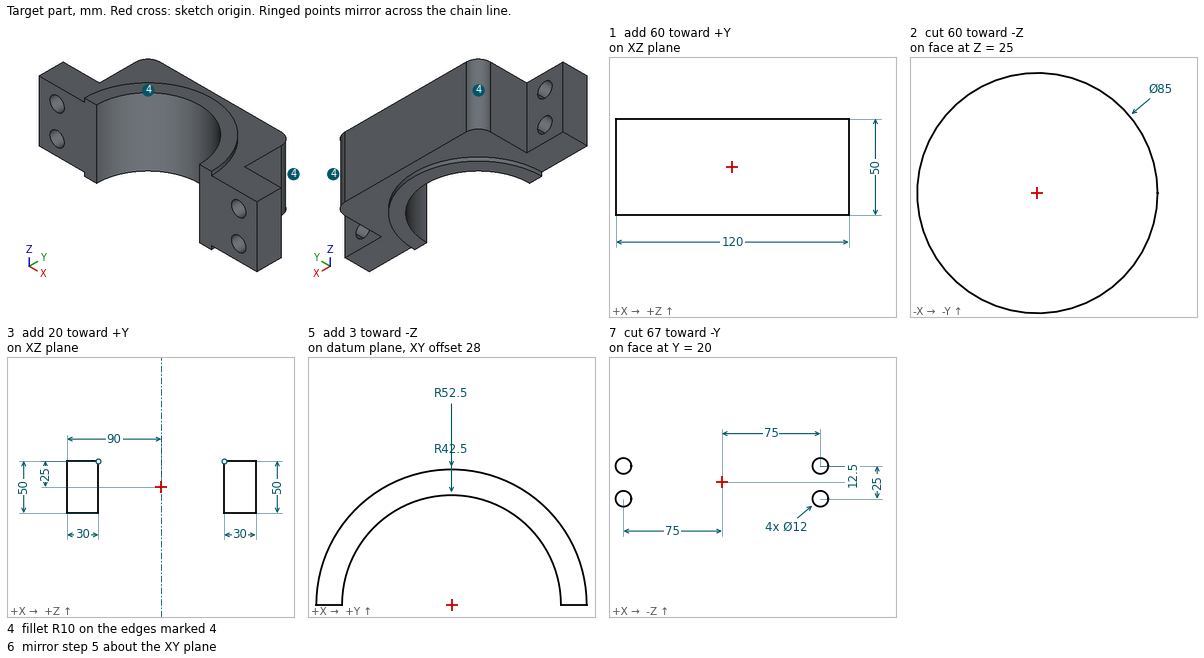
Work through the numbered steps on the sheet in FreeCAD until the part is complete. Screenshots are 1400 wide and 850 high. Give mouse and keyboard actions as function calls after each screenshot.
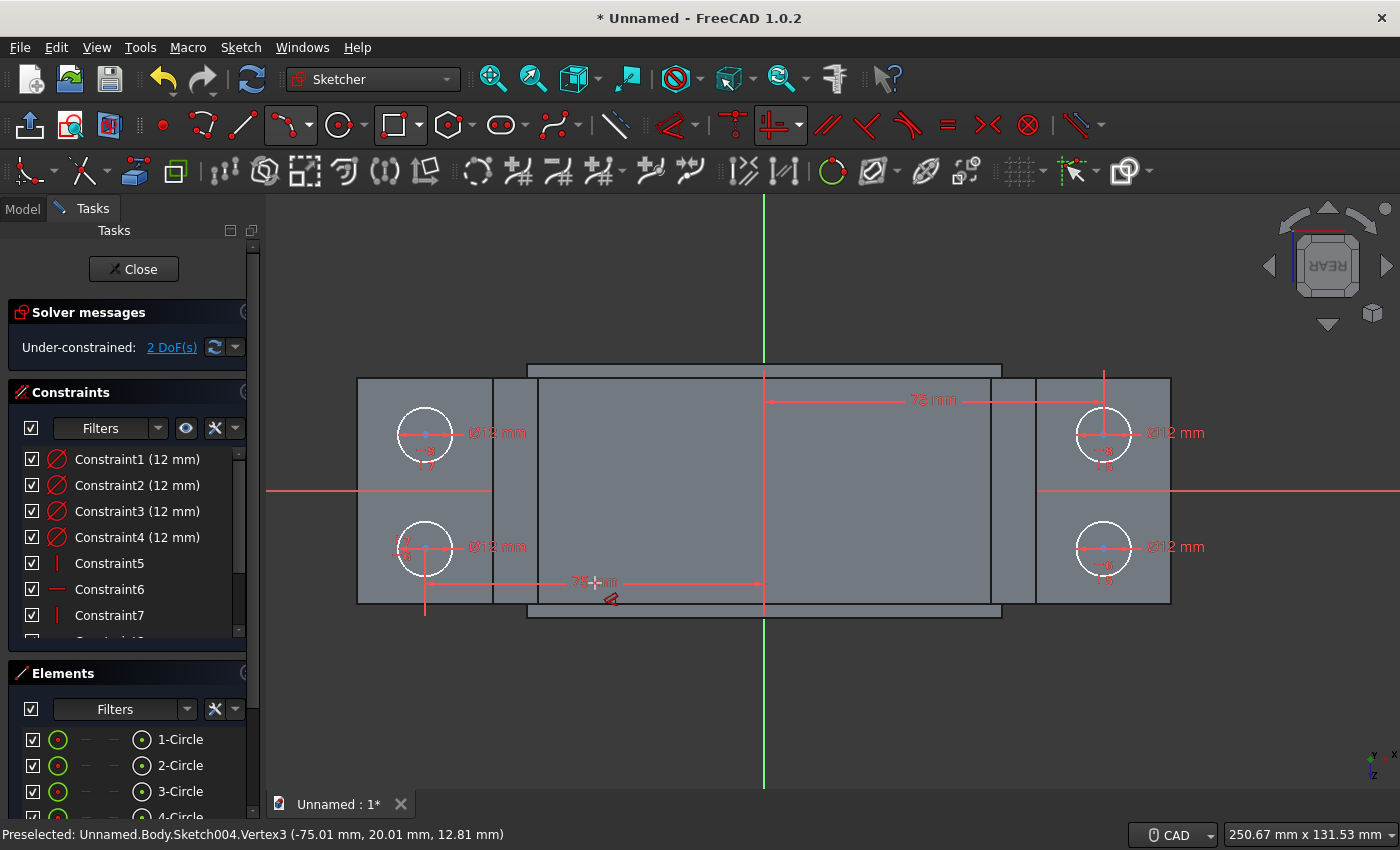
click(1104, 435)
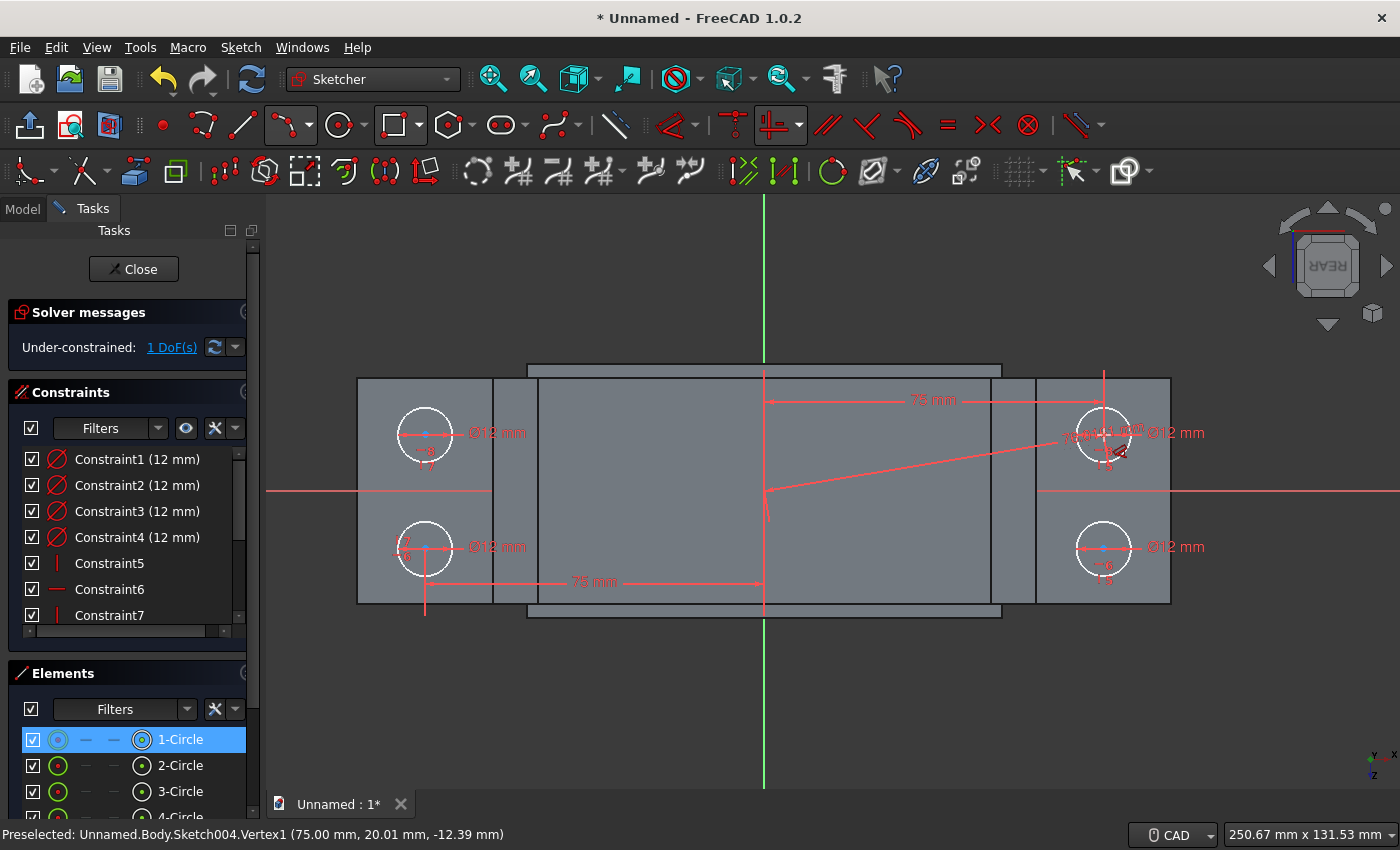
click(1104, 549)
click(1138, 466)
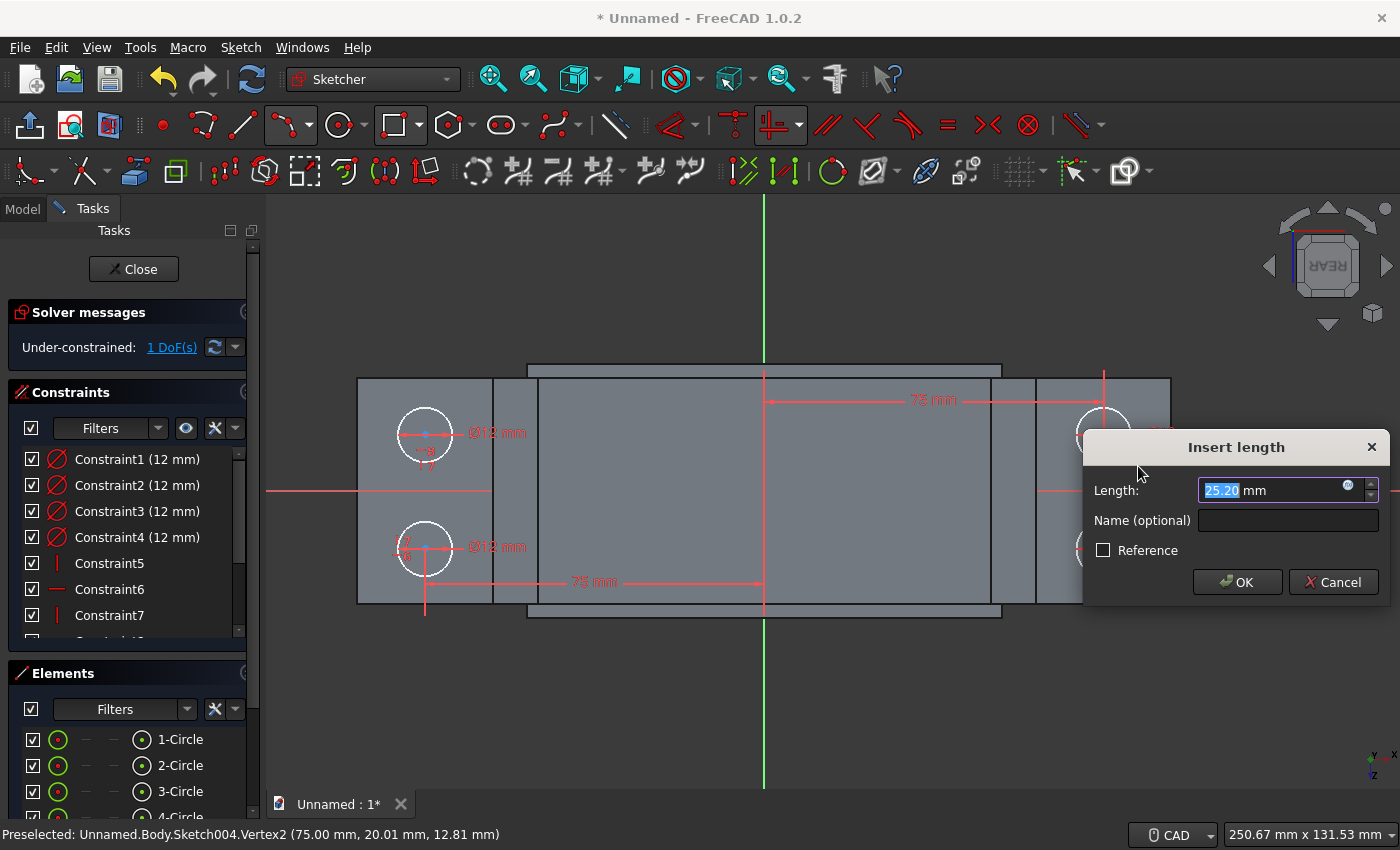
text(25)
key(Return)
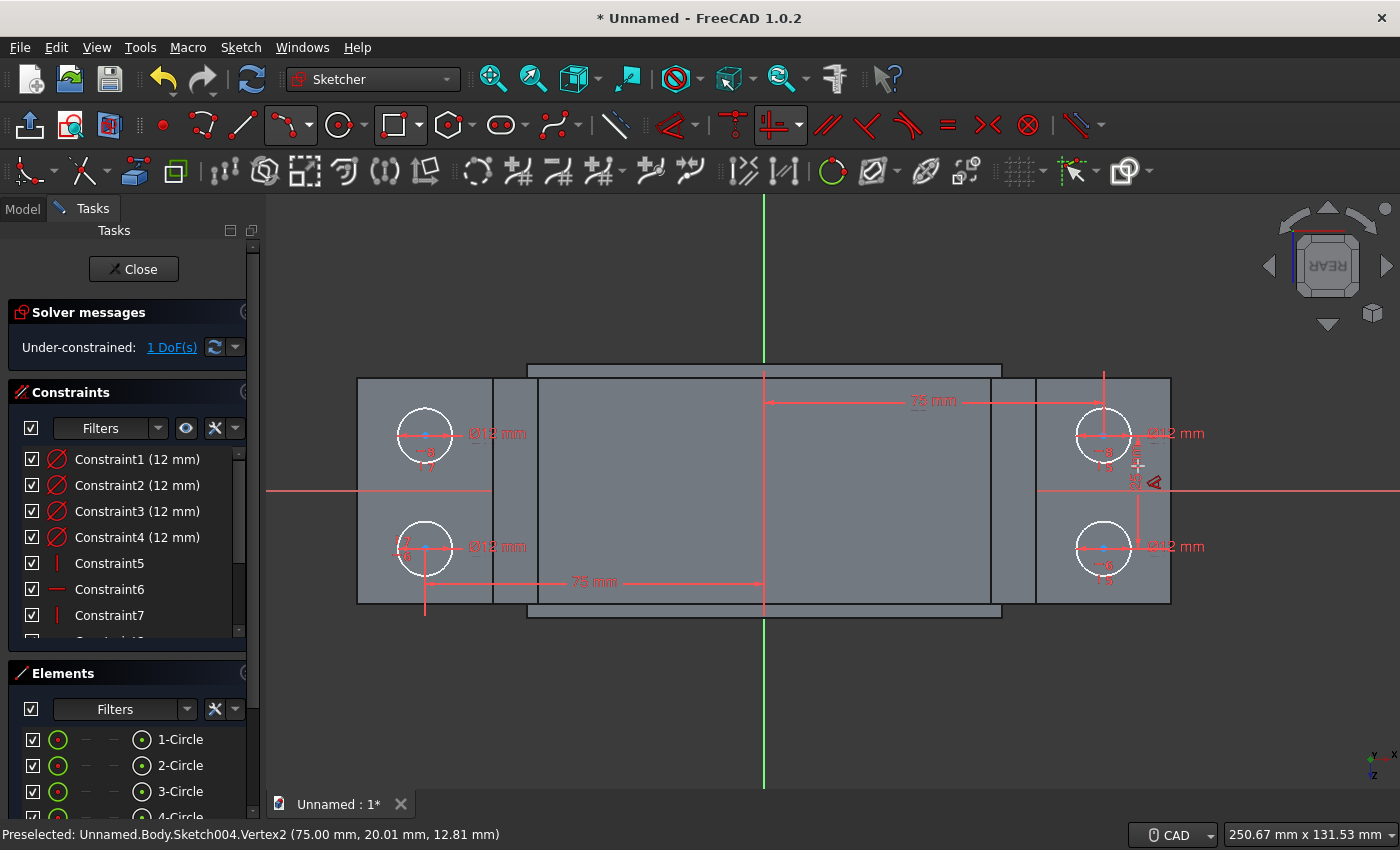
click(1104, 436)
click(730, 463)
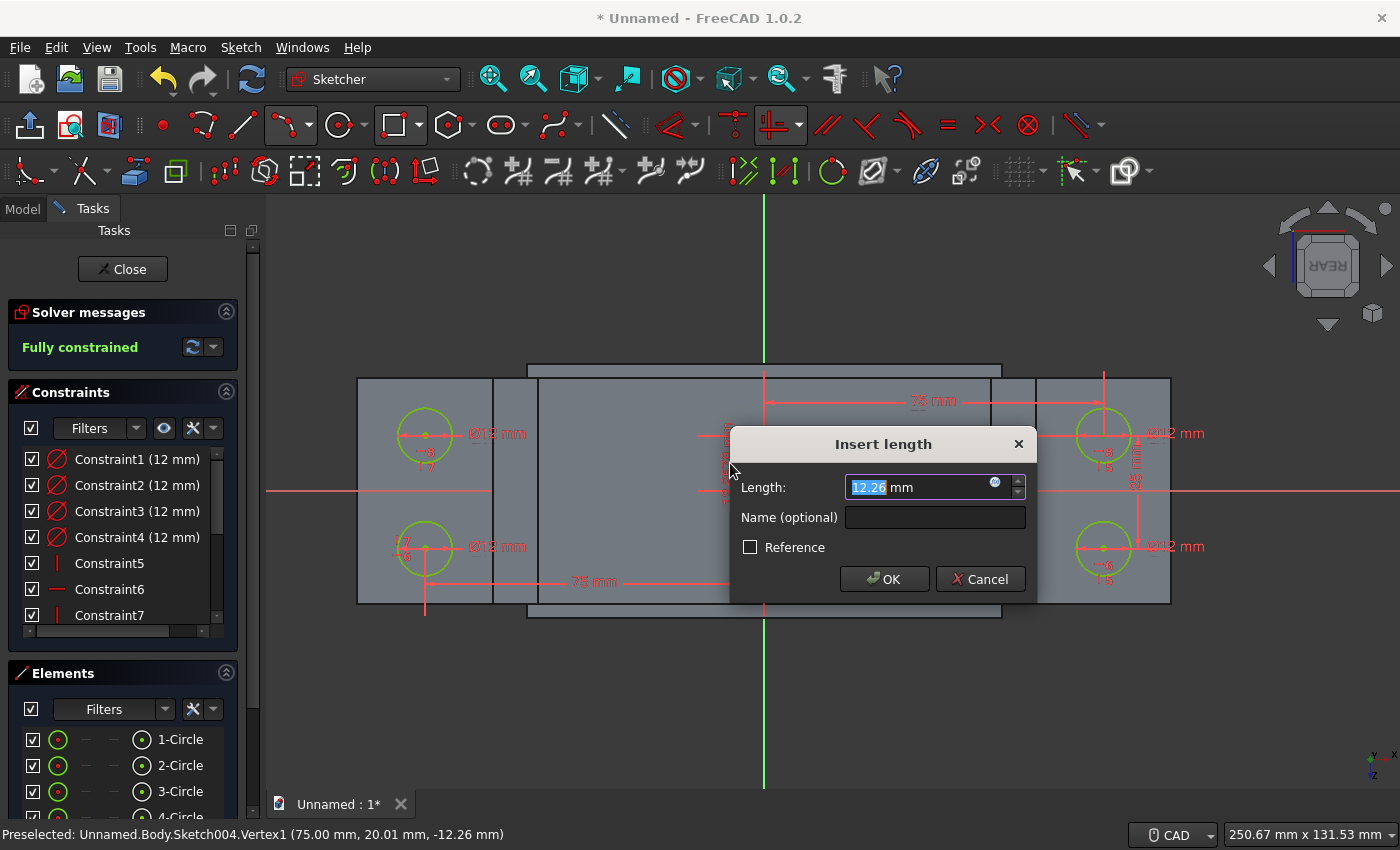
text(12.5)
key(Return)
key(Escape)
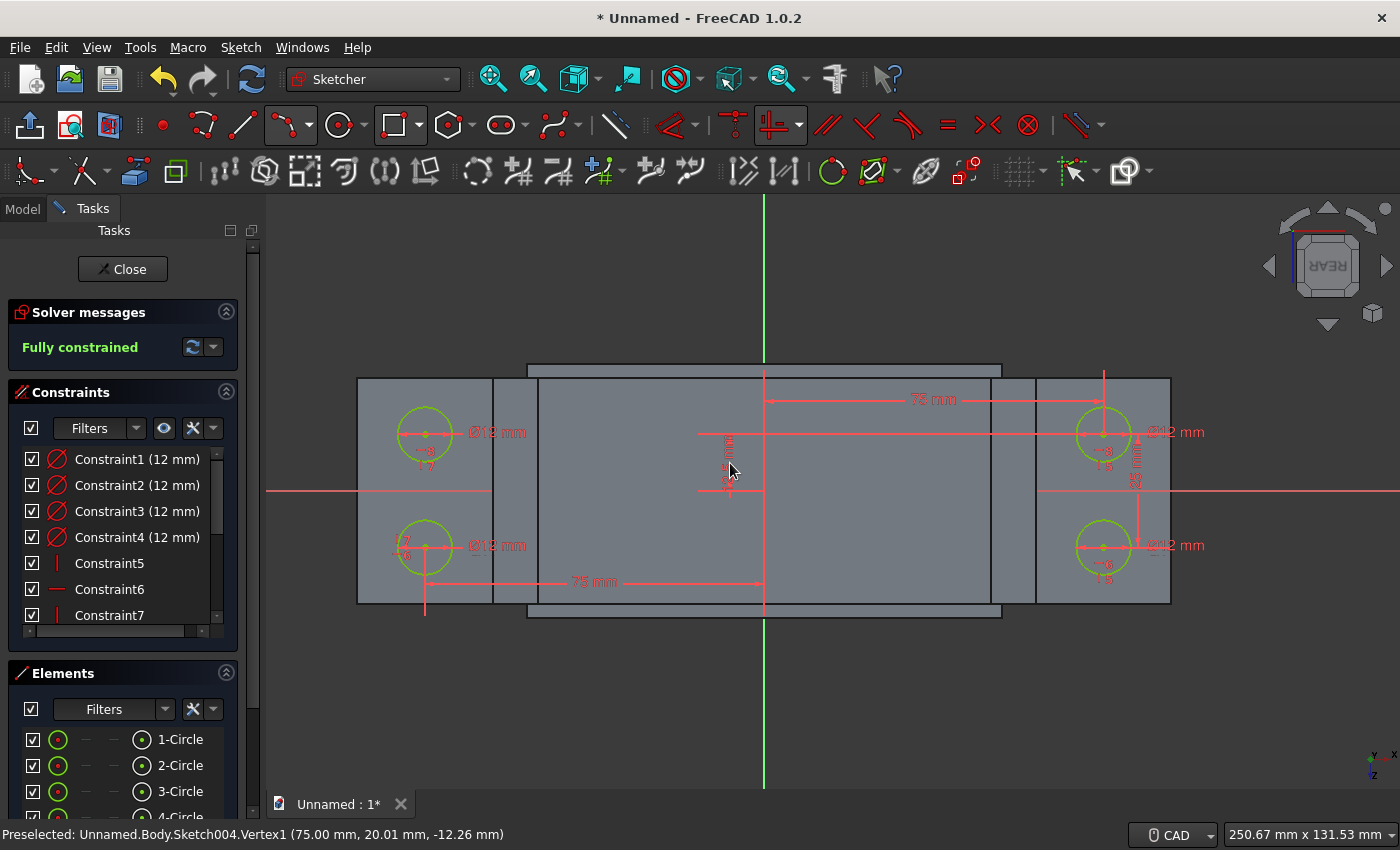
click(123, 269)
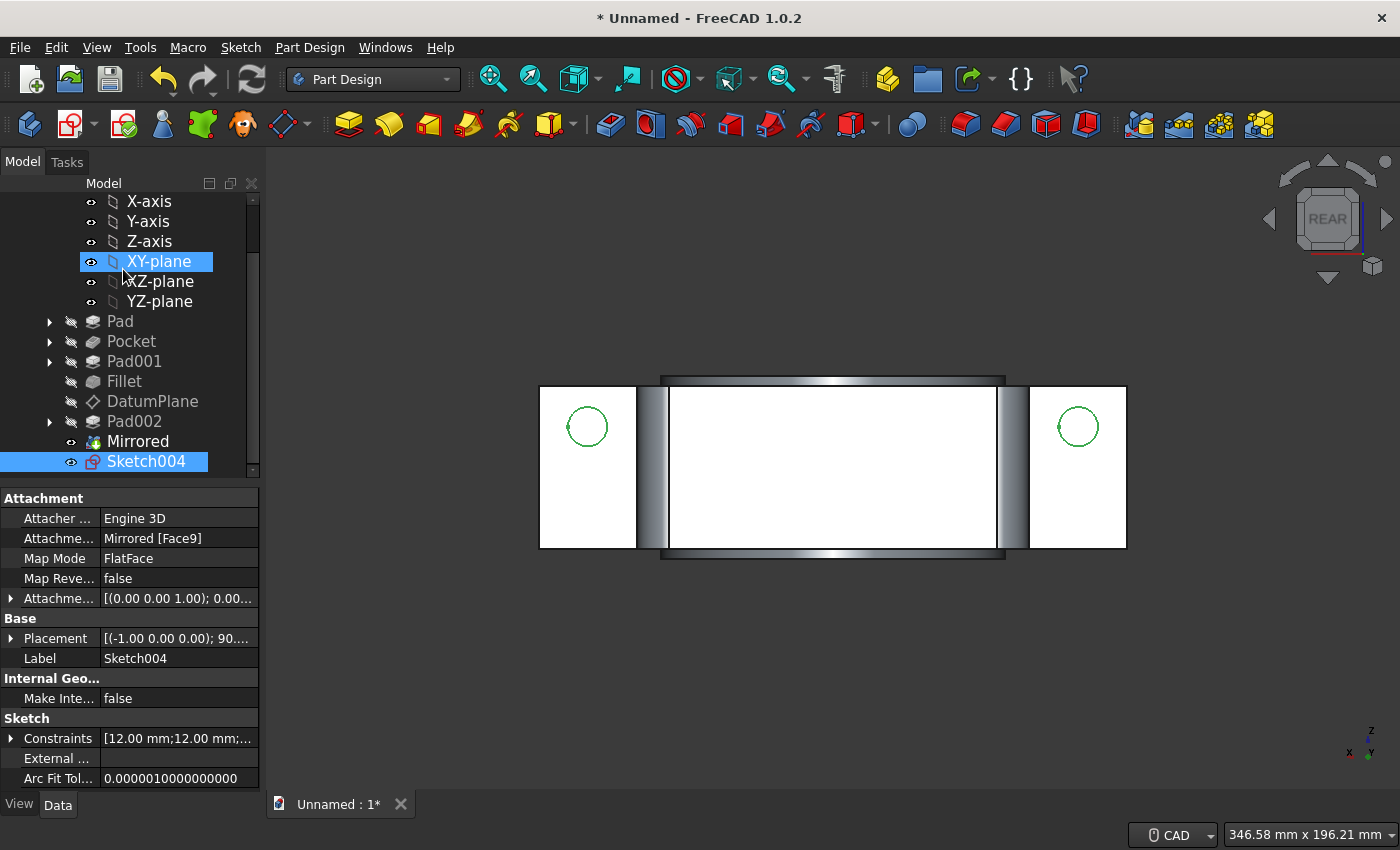
click(612, 124)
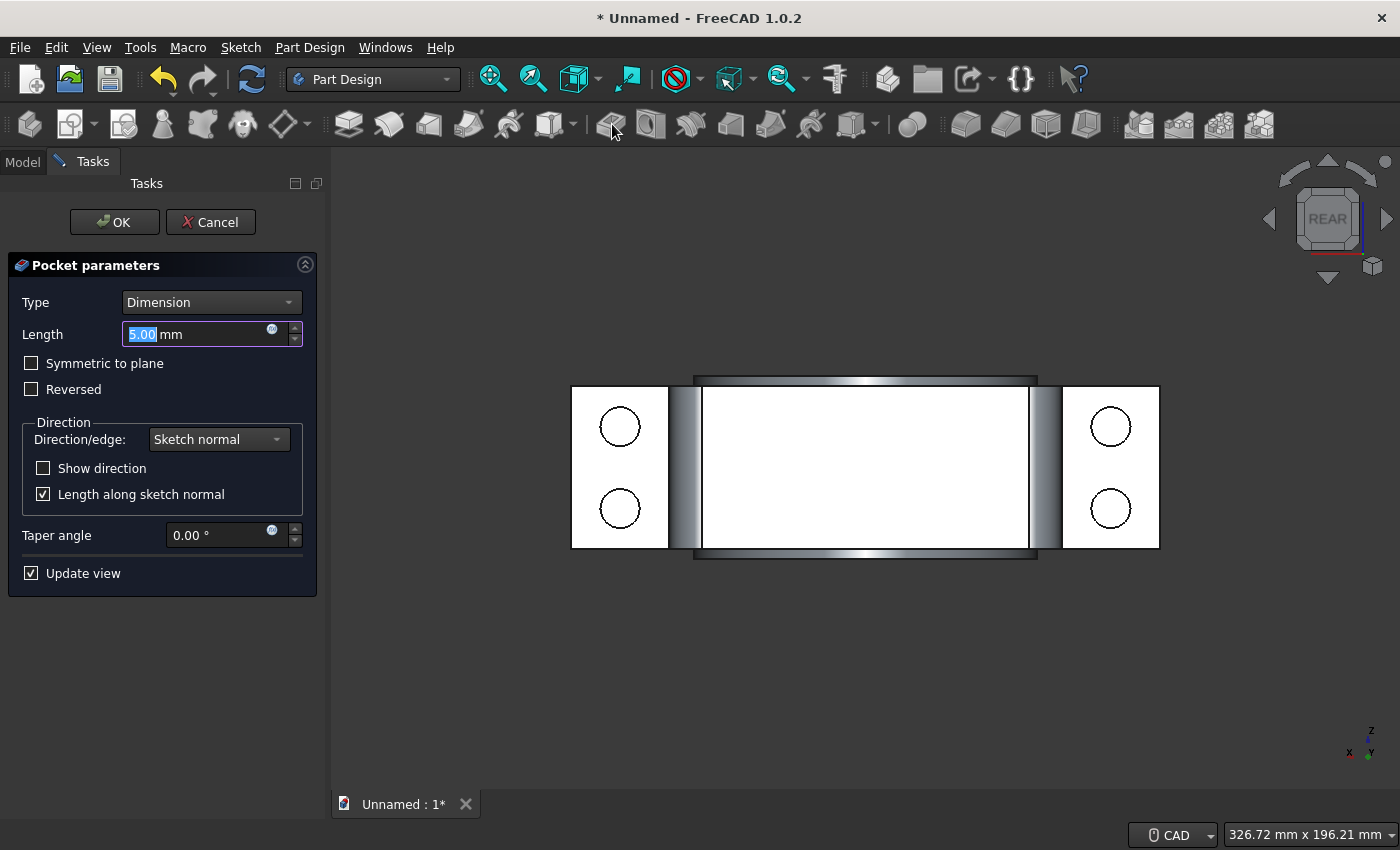
text(67)
key(Tab)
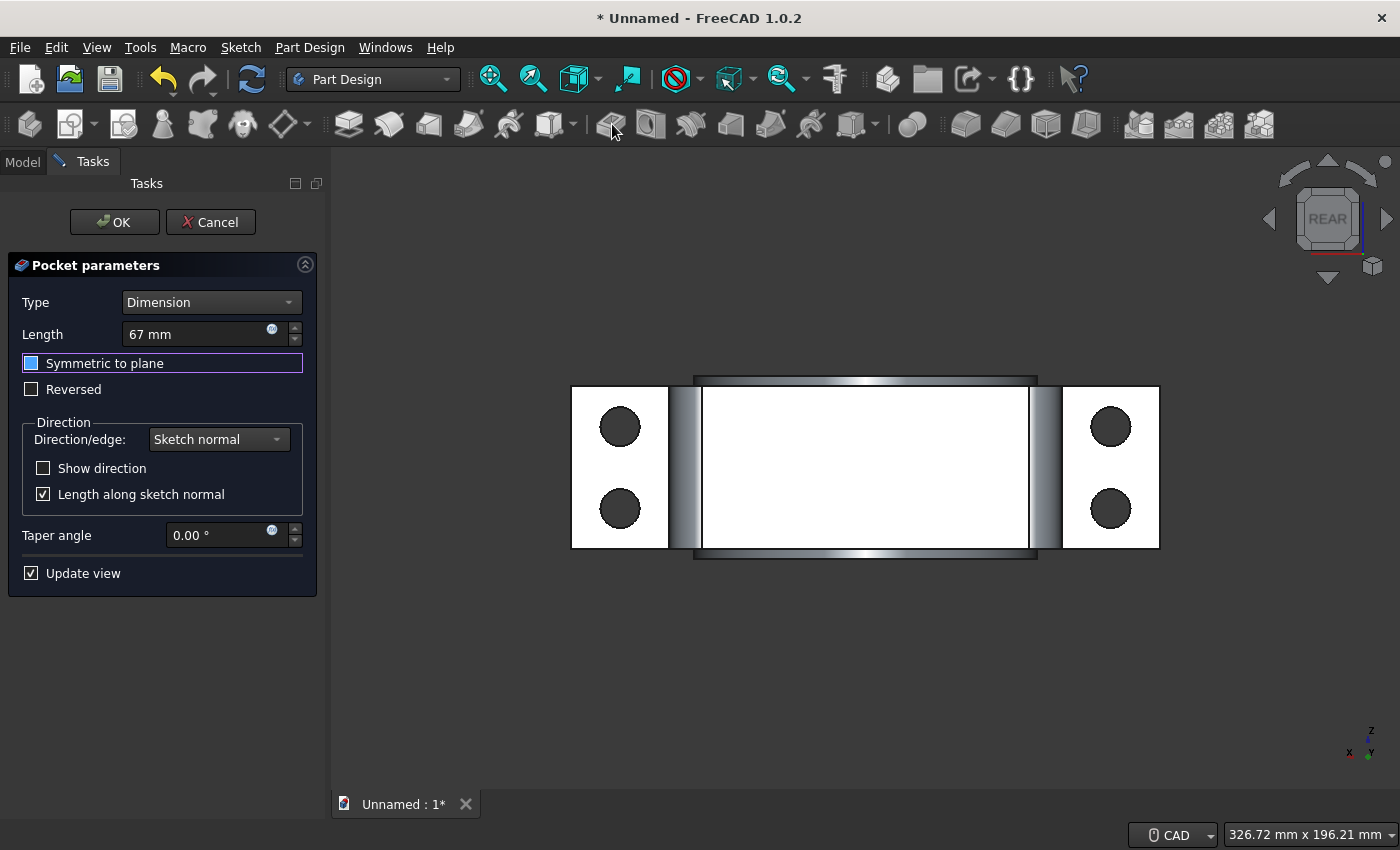
click(115, 222)